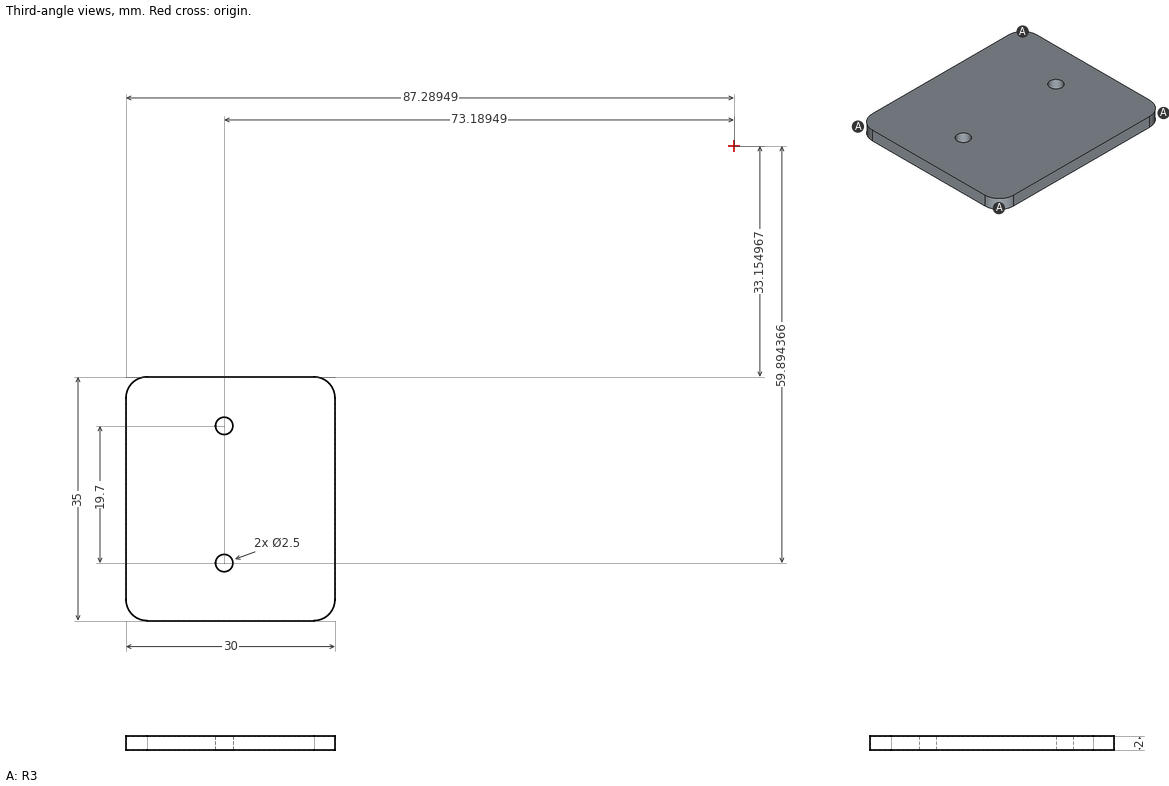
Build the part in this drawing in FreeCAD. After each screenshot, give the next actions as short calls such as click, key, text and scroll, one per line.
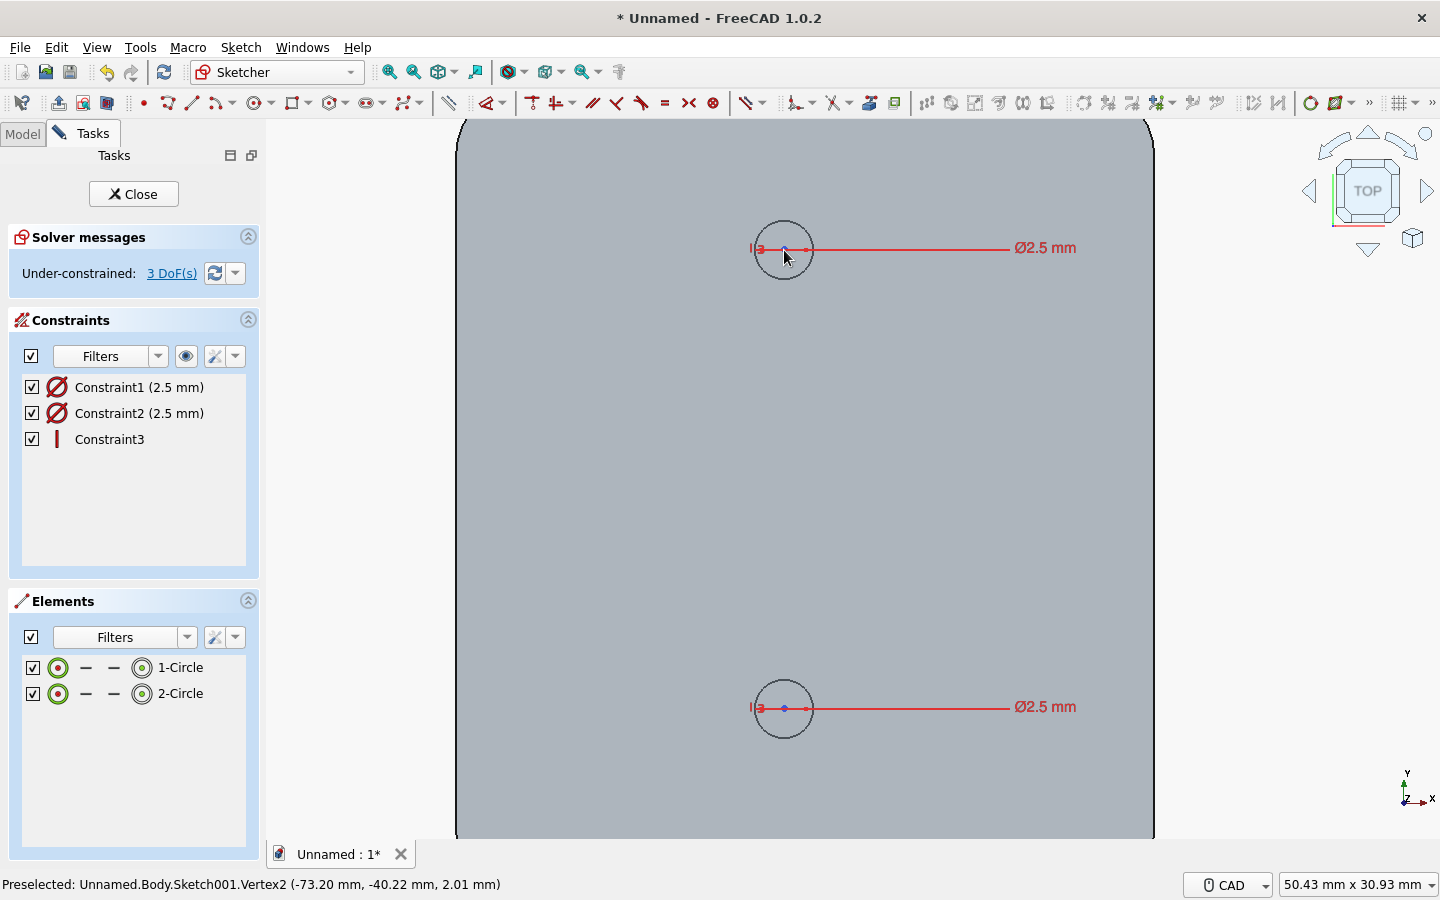
click(784, 709)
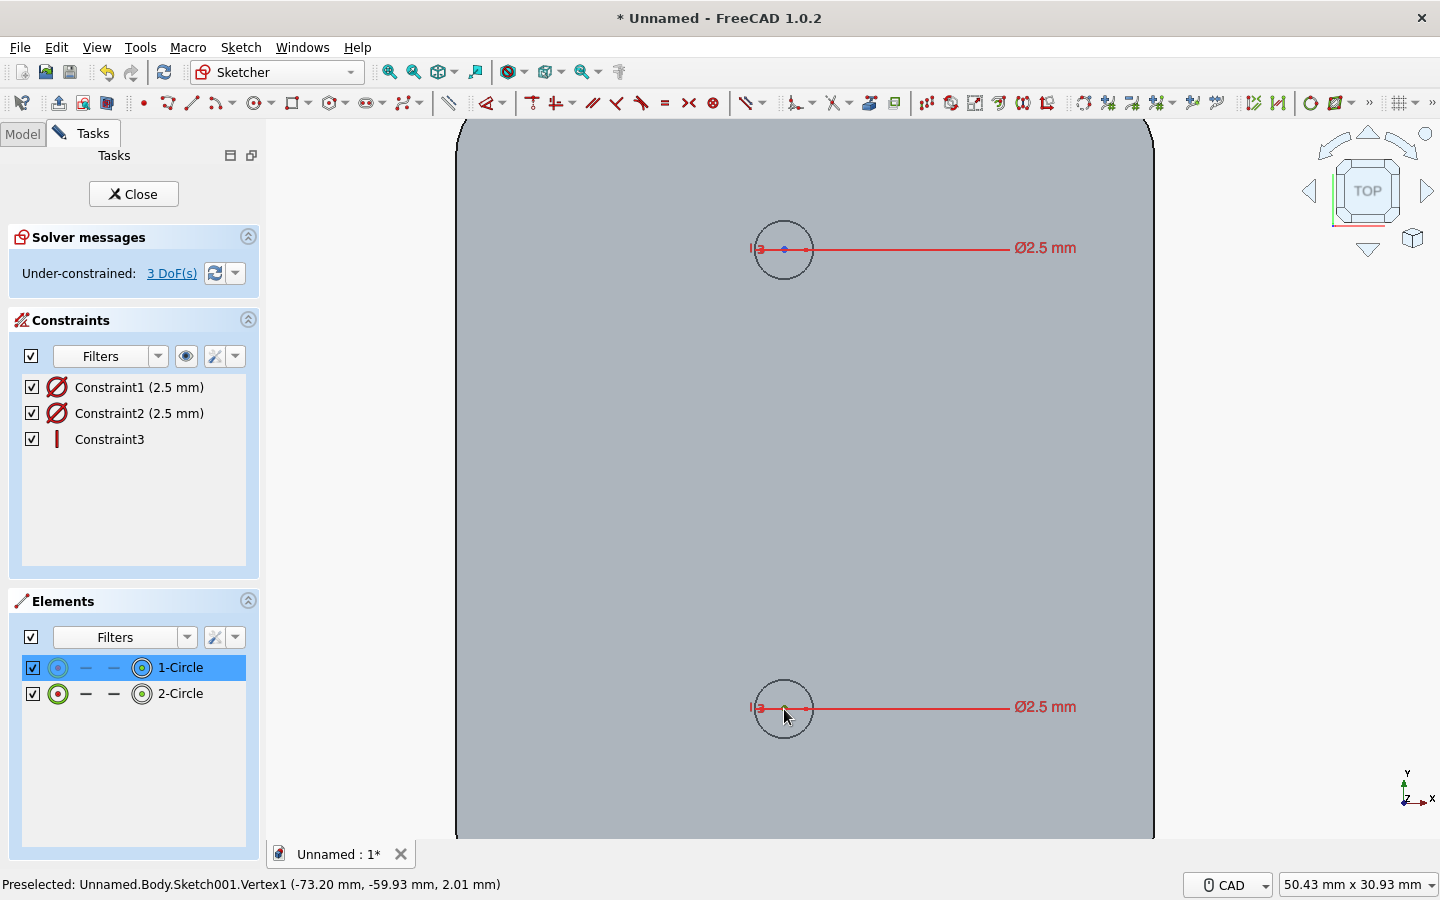
click(784, 250)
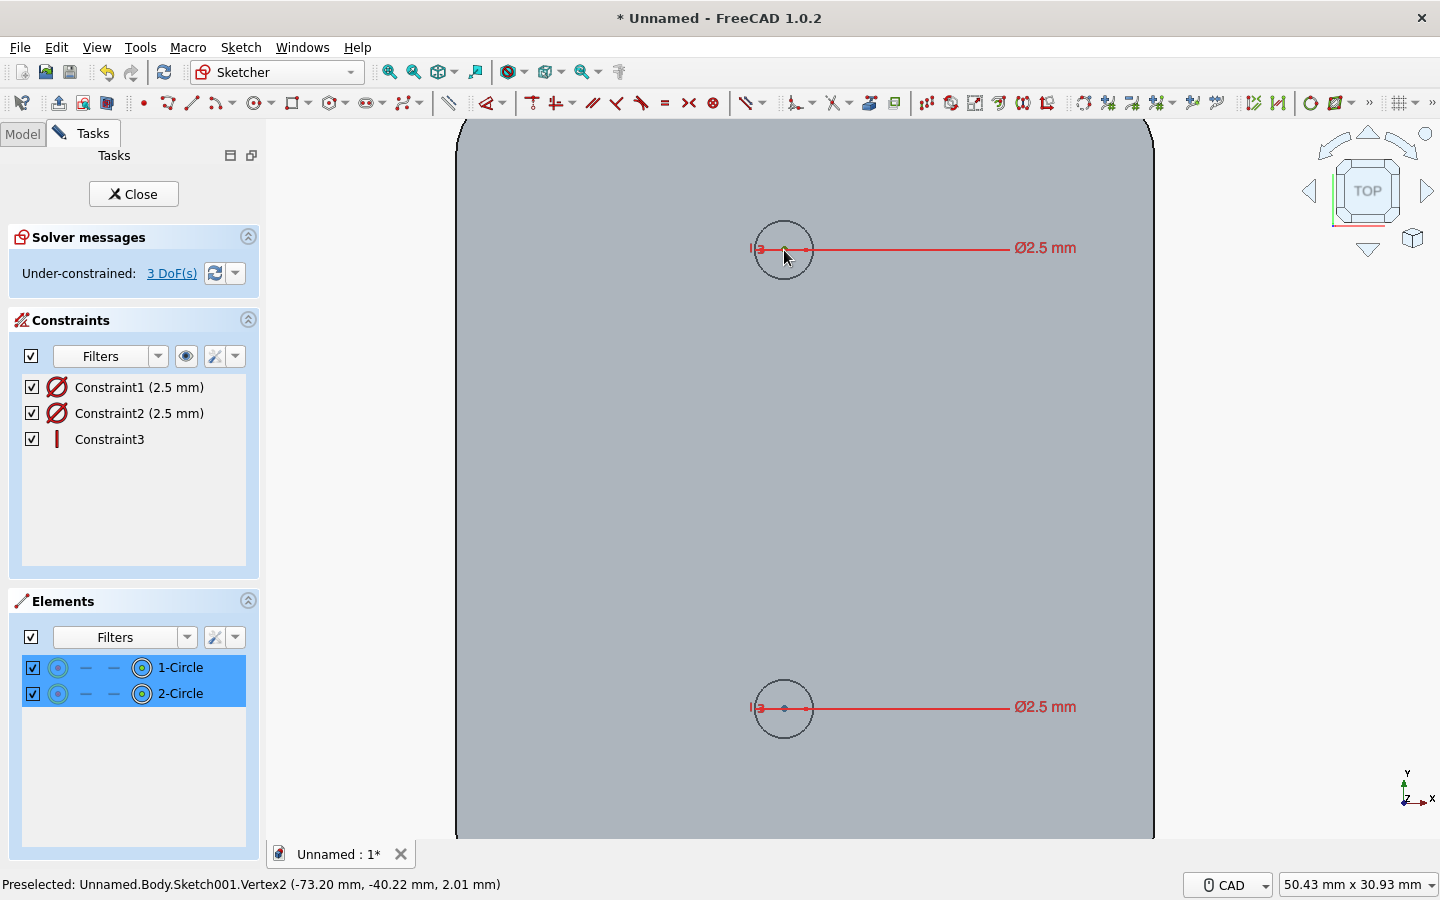
click(504, 104)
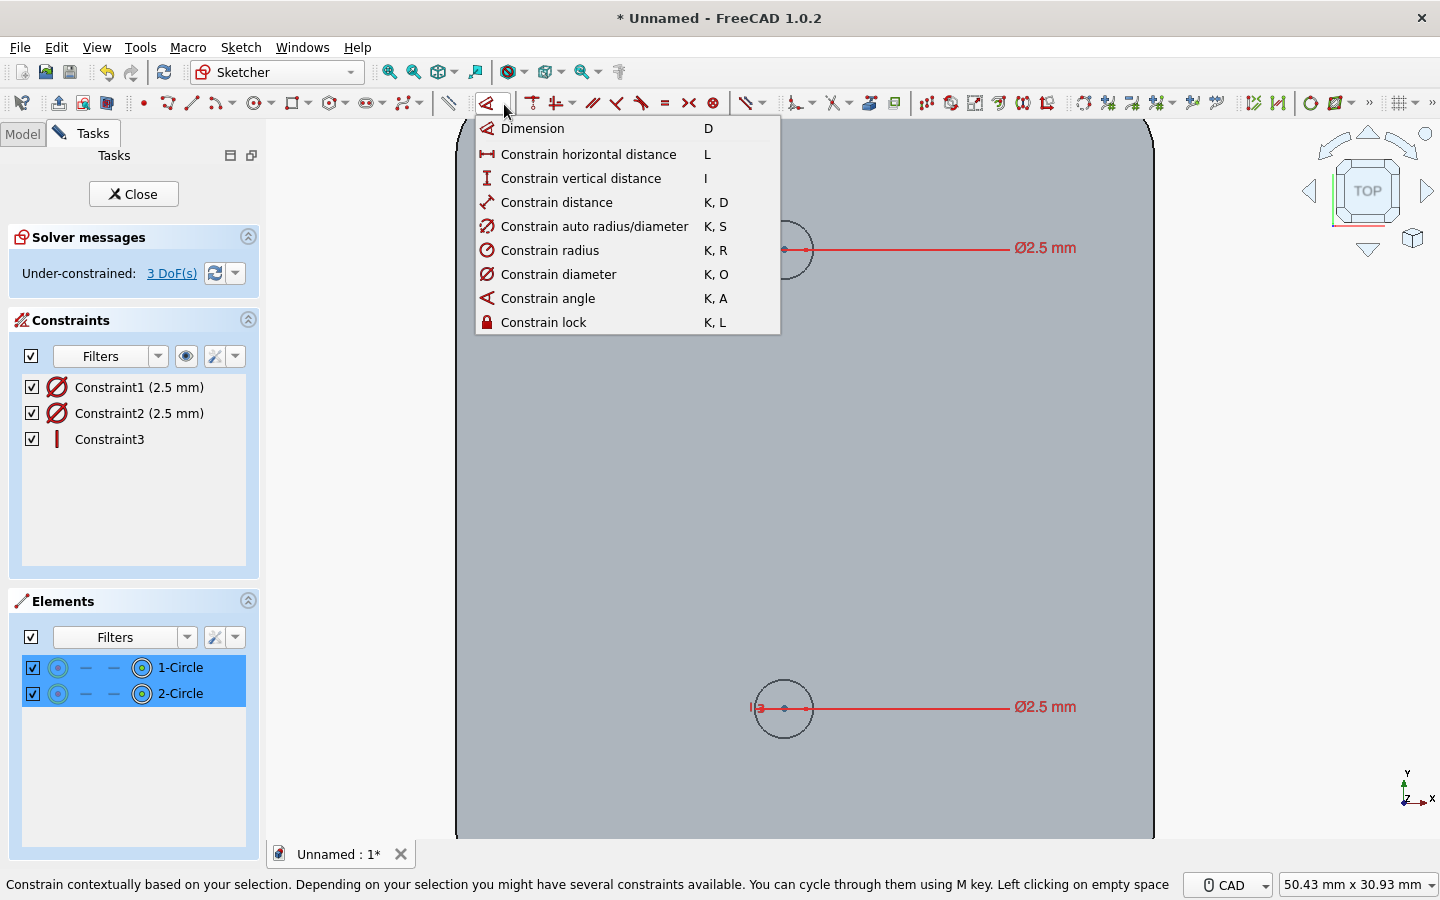
click(628, 178)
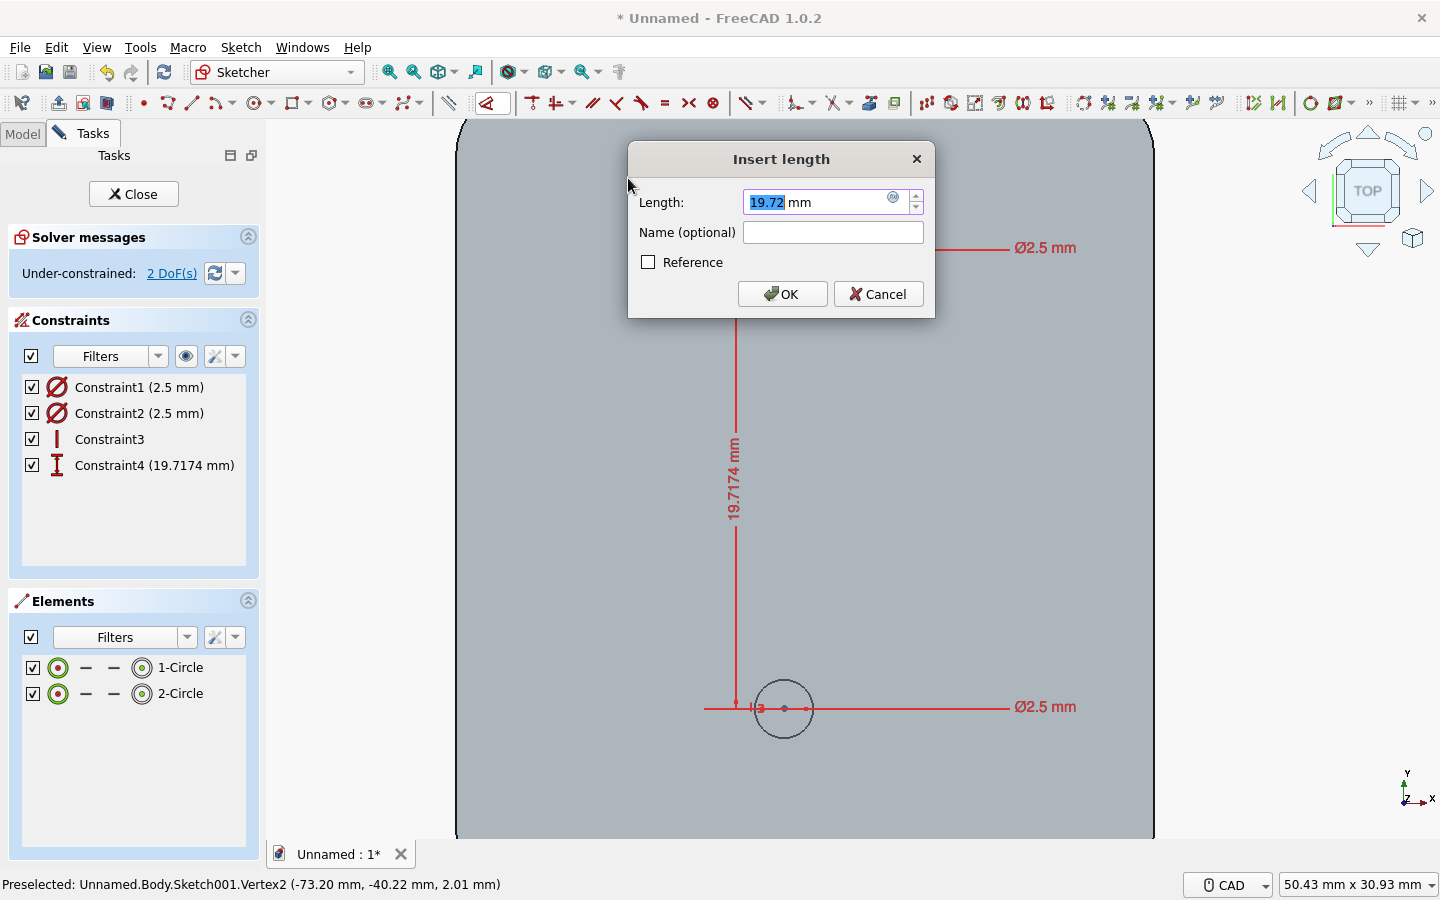
text(19.7)
key(Return)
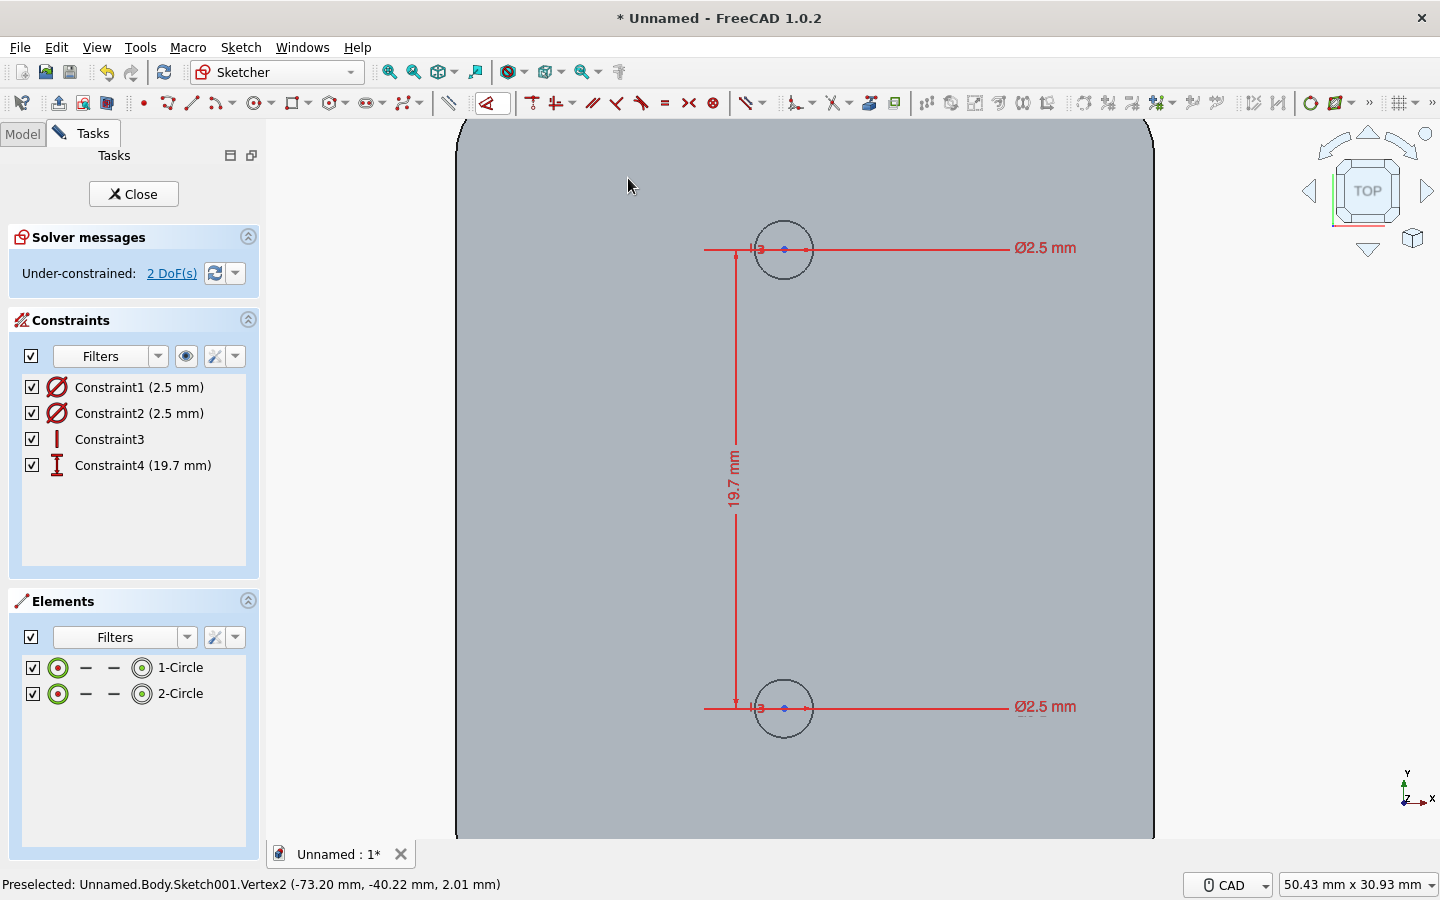
click(784, 709)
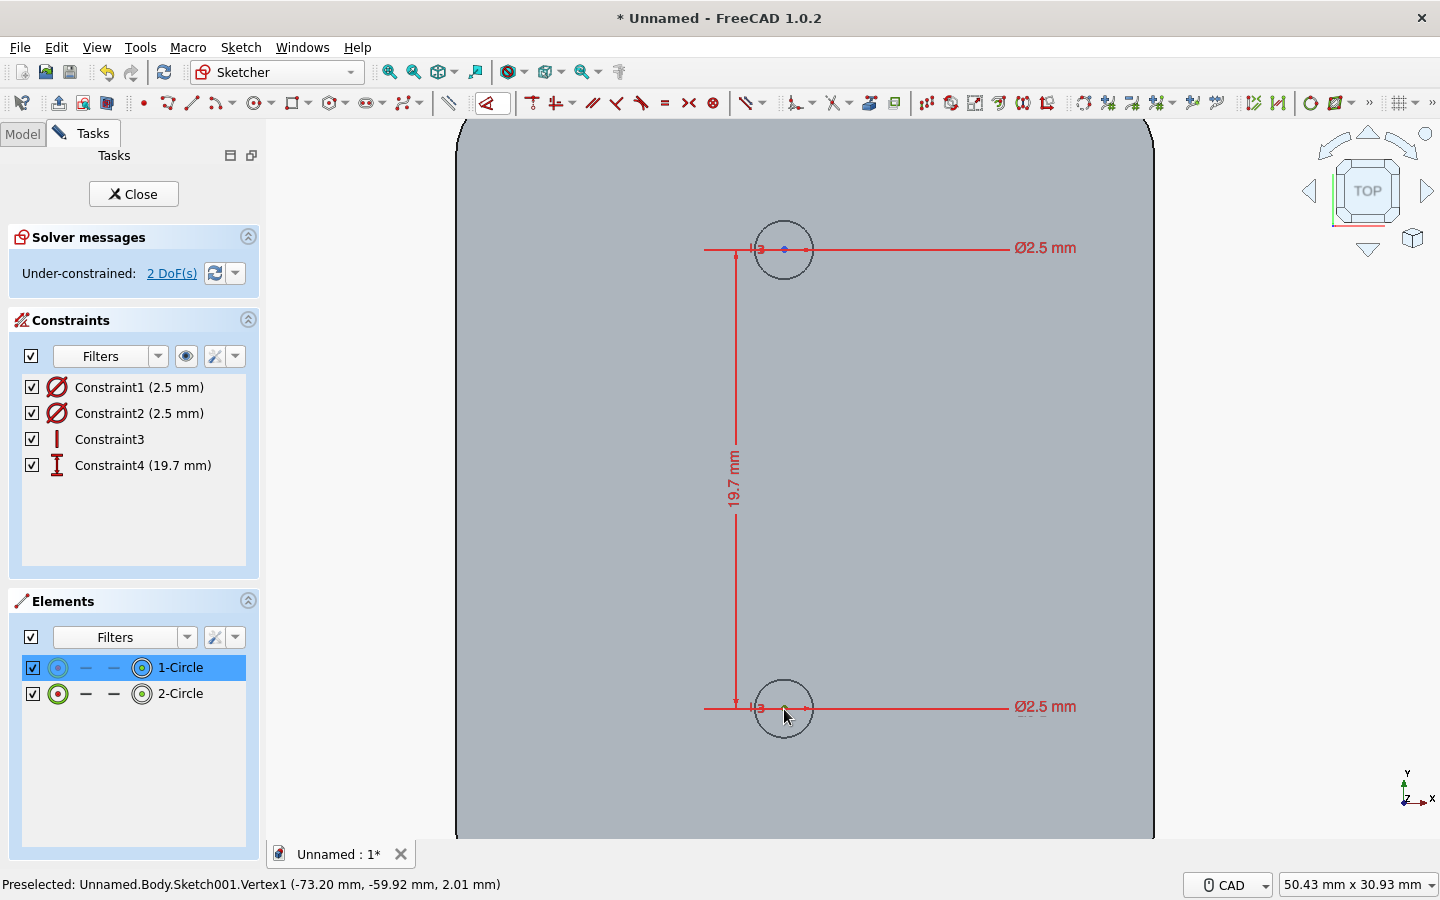
click(504, 104)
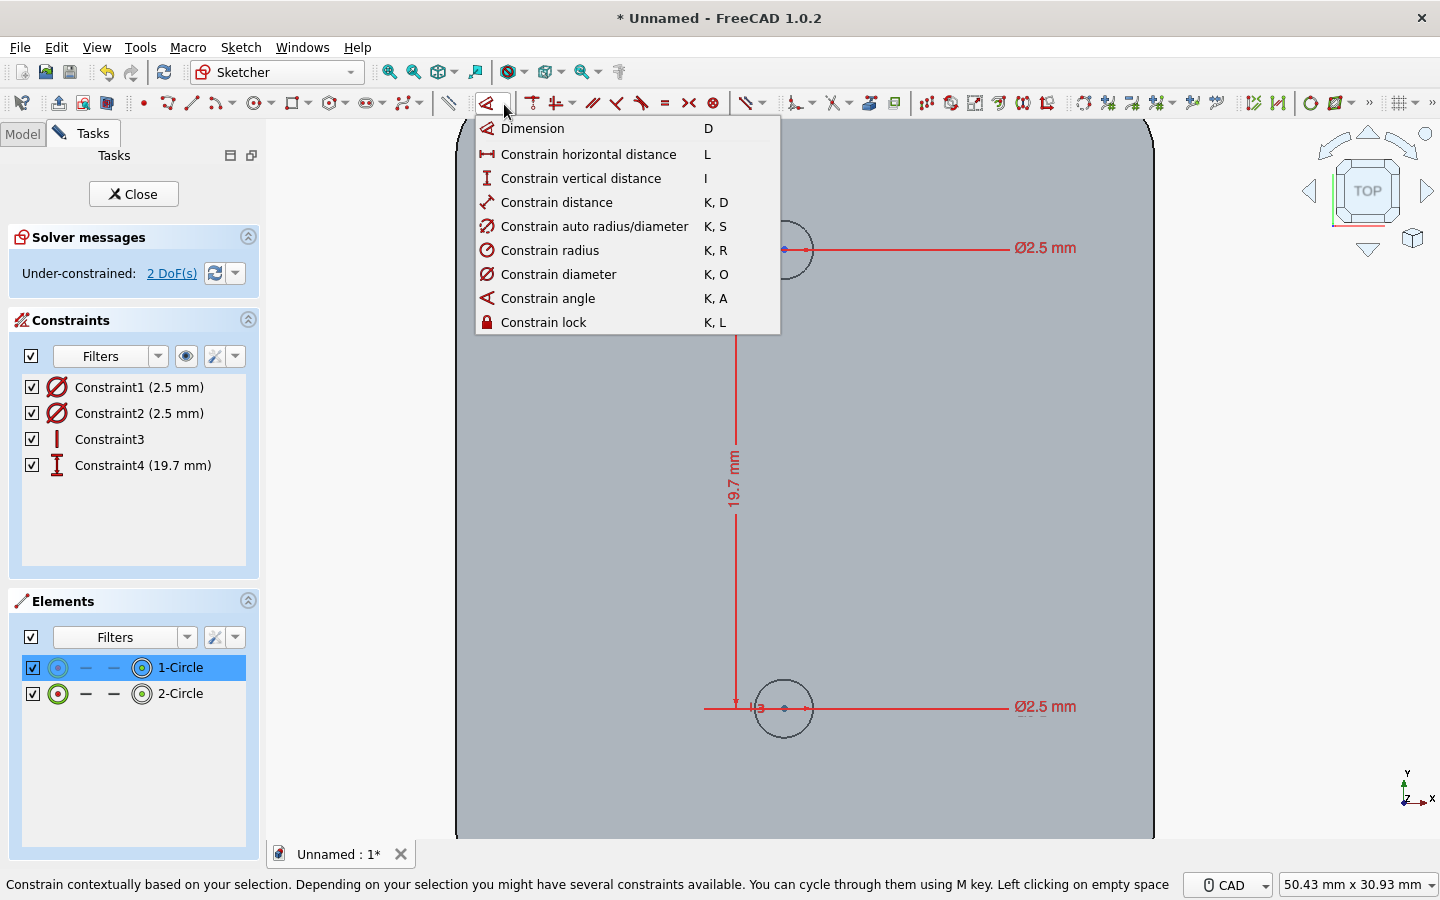
click(628, 154)